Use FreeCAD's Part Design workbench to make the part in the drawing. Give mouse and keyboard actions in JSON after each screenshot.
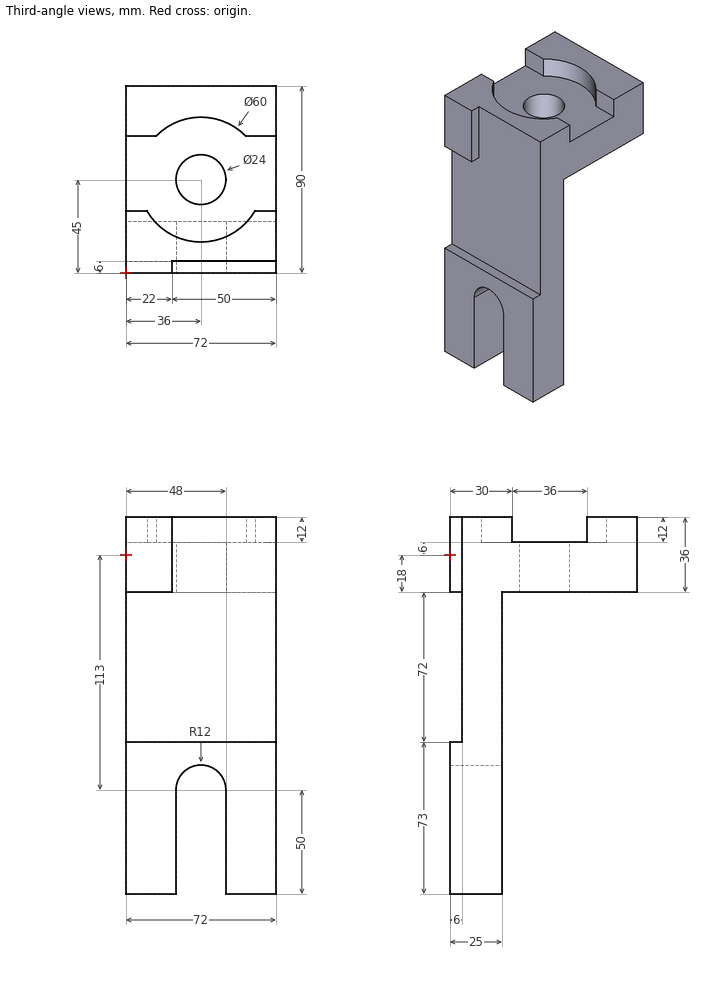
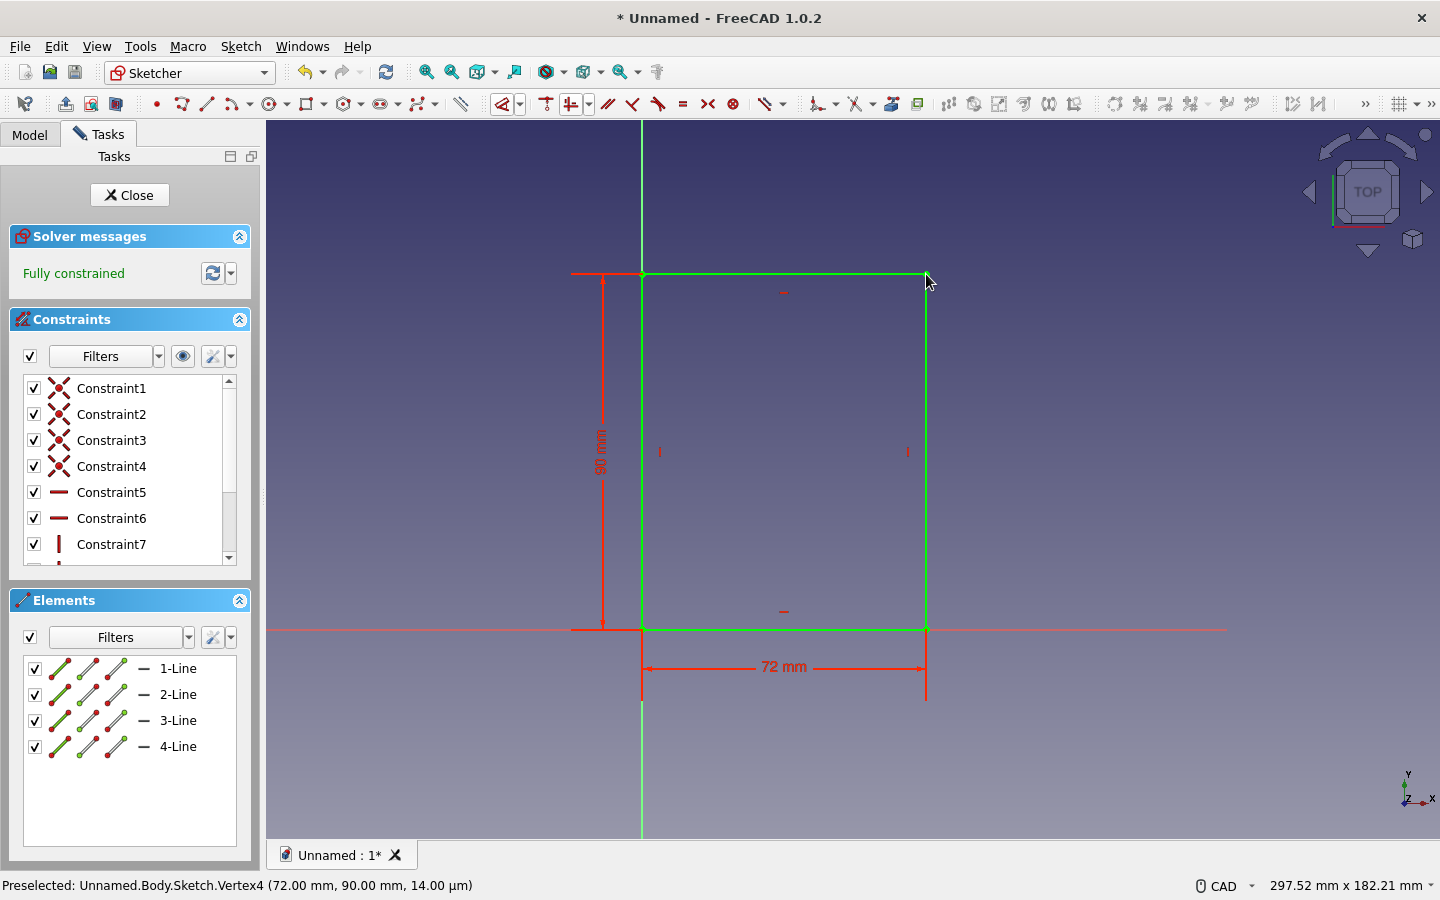
{"action": "left_click", "coordinate": [130, 195]}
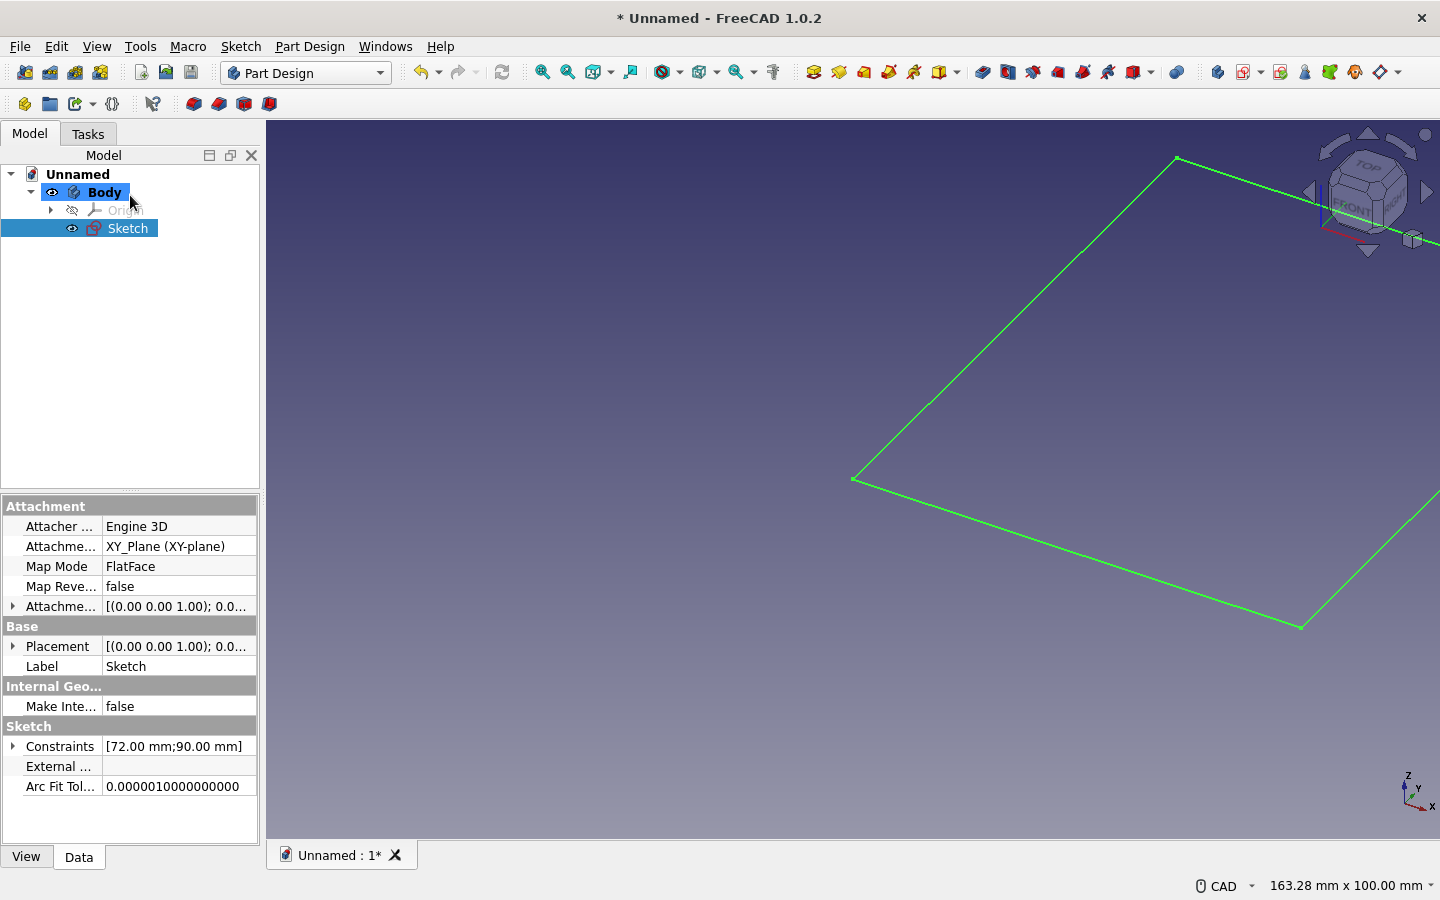
{"action": "left_click", "coordinate": [814, 72]}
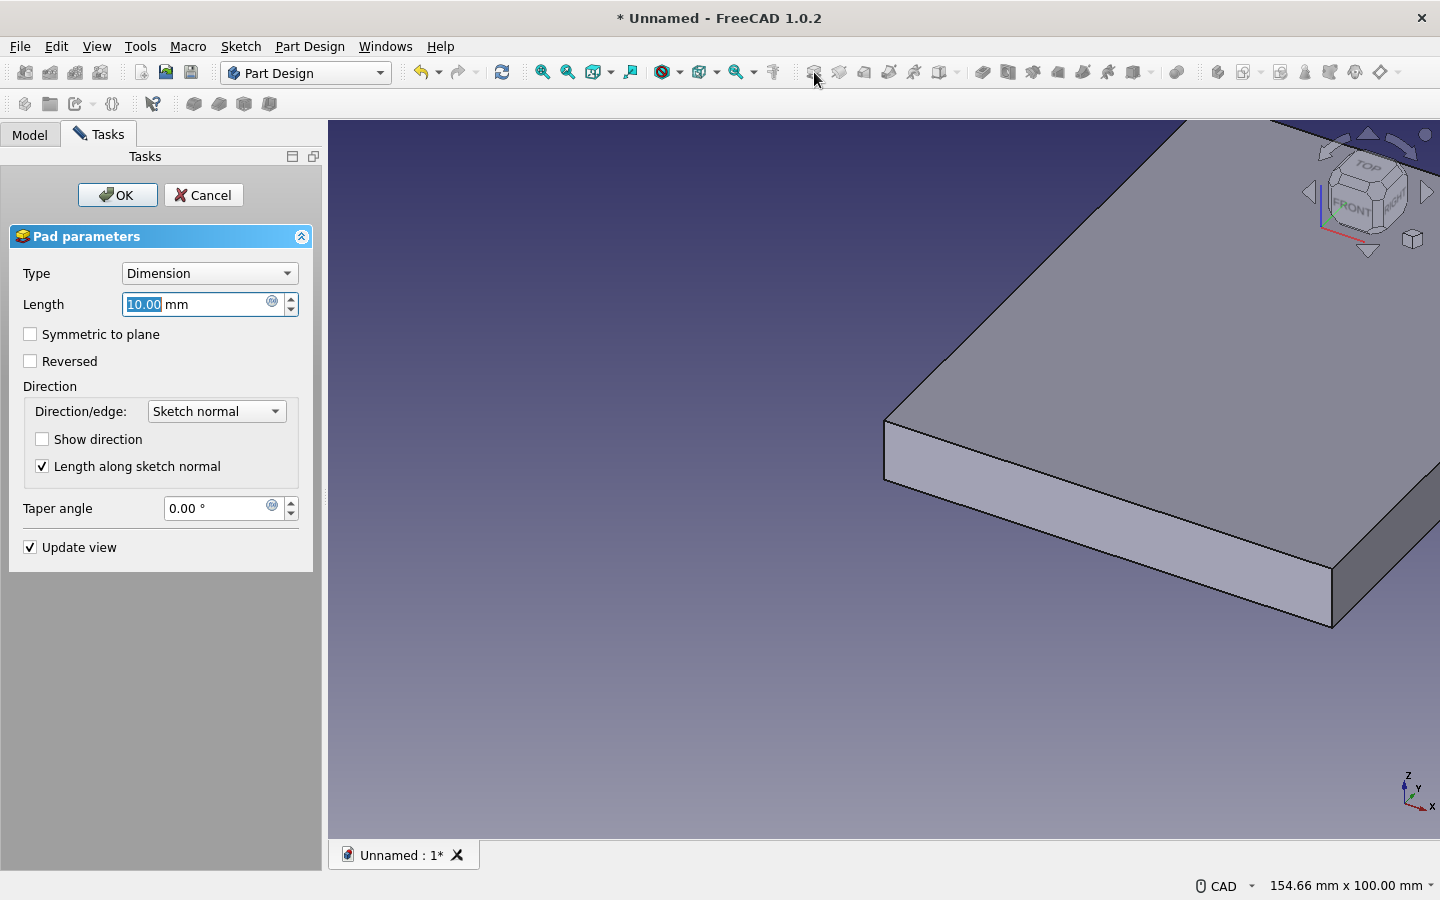
{"action": "type", "text": "36"}
{"action": "key", "text": "Tab"}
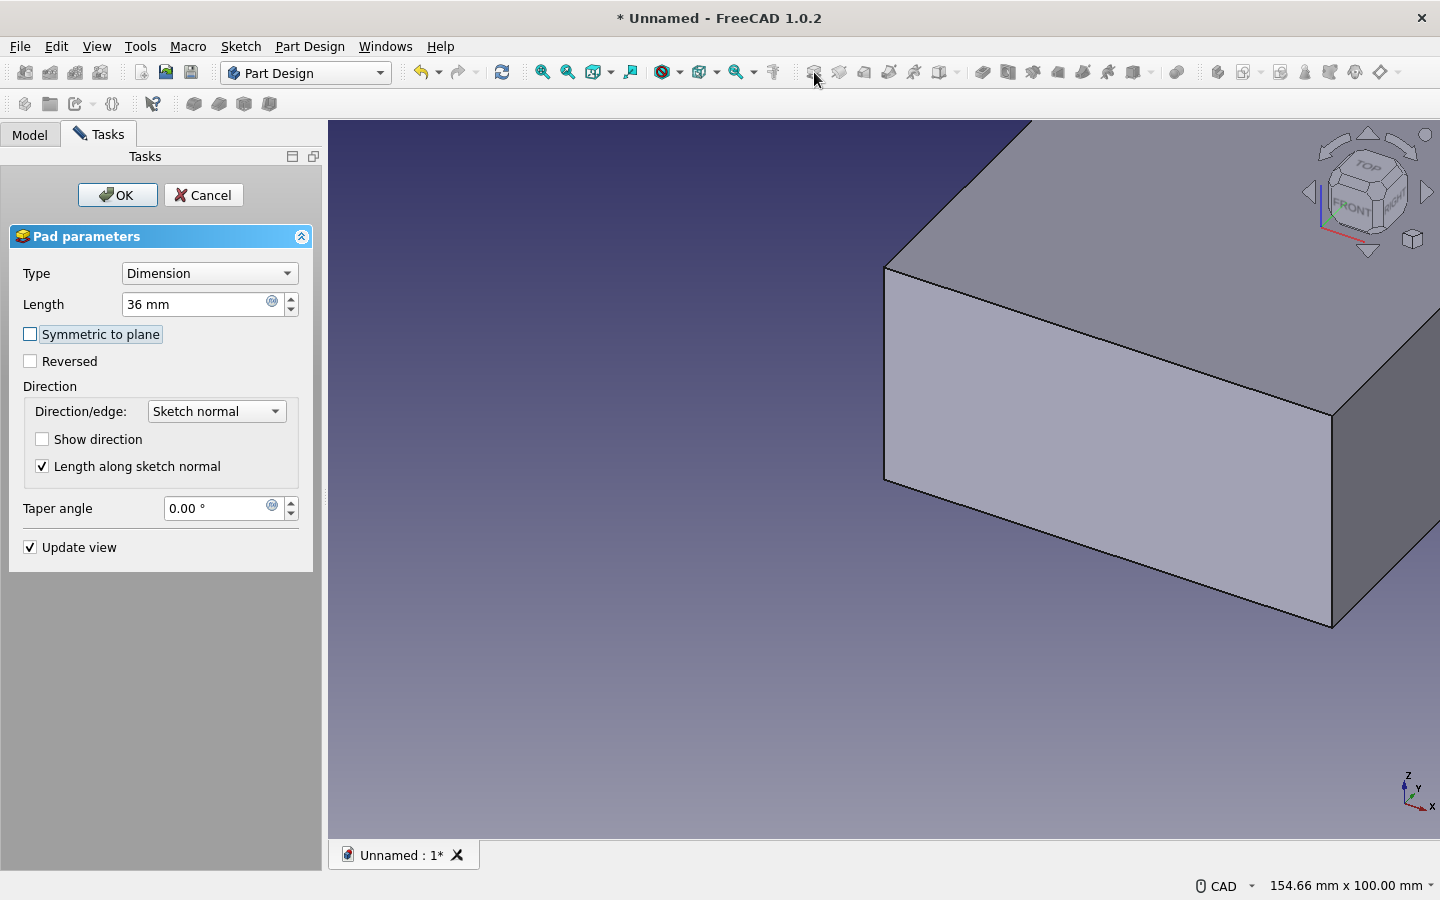
{"action": "left_click", "coordinate": [31, 334]}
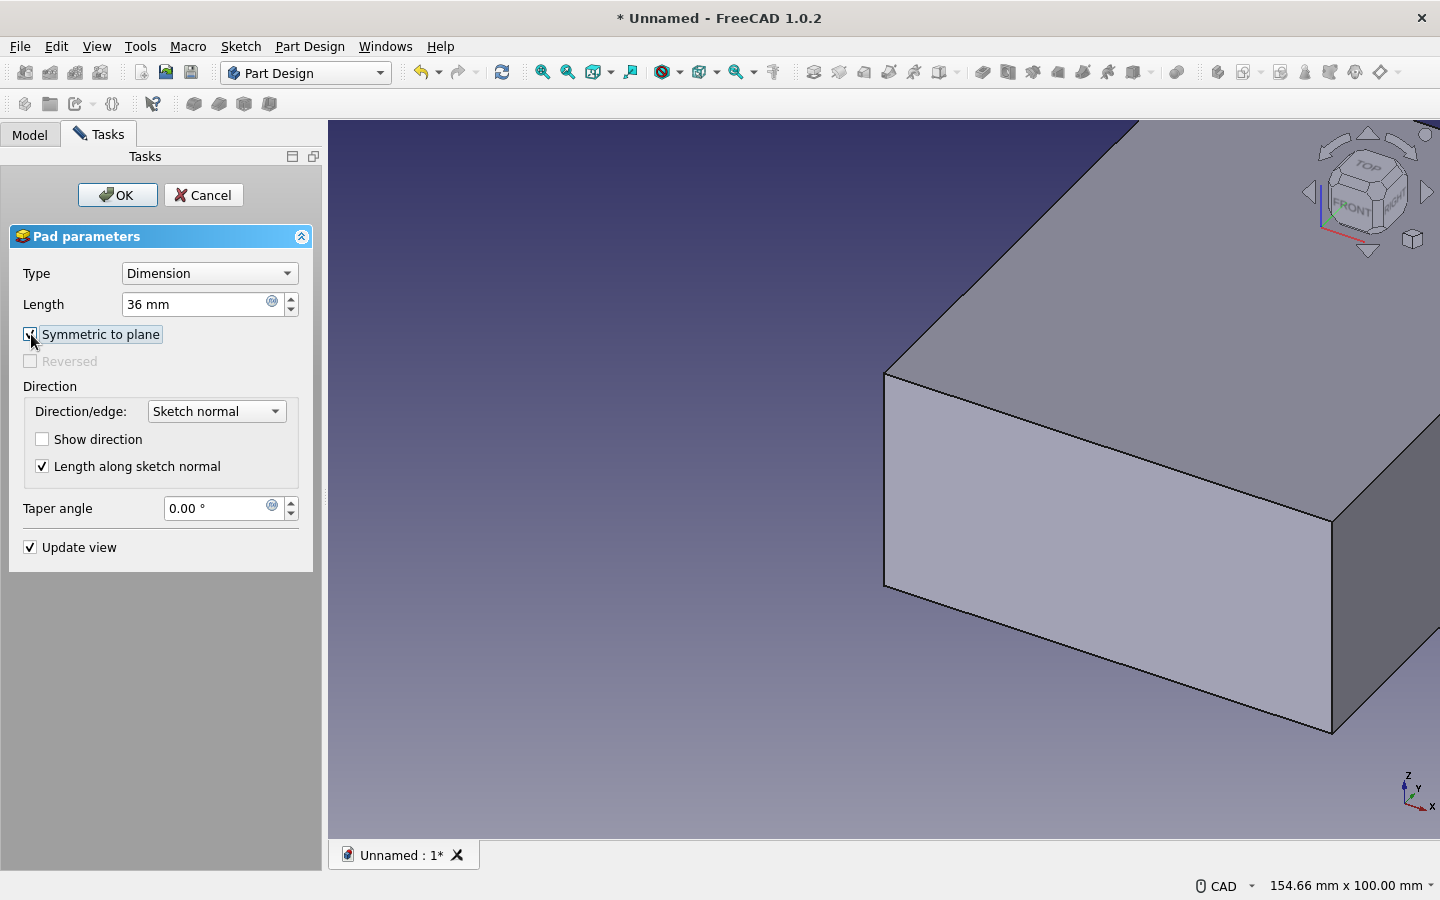
{"action": "left_click", "coordinate": [118, 195]}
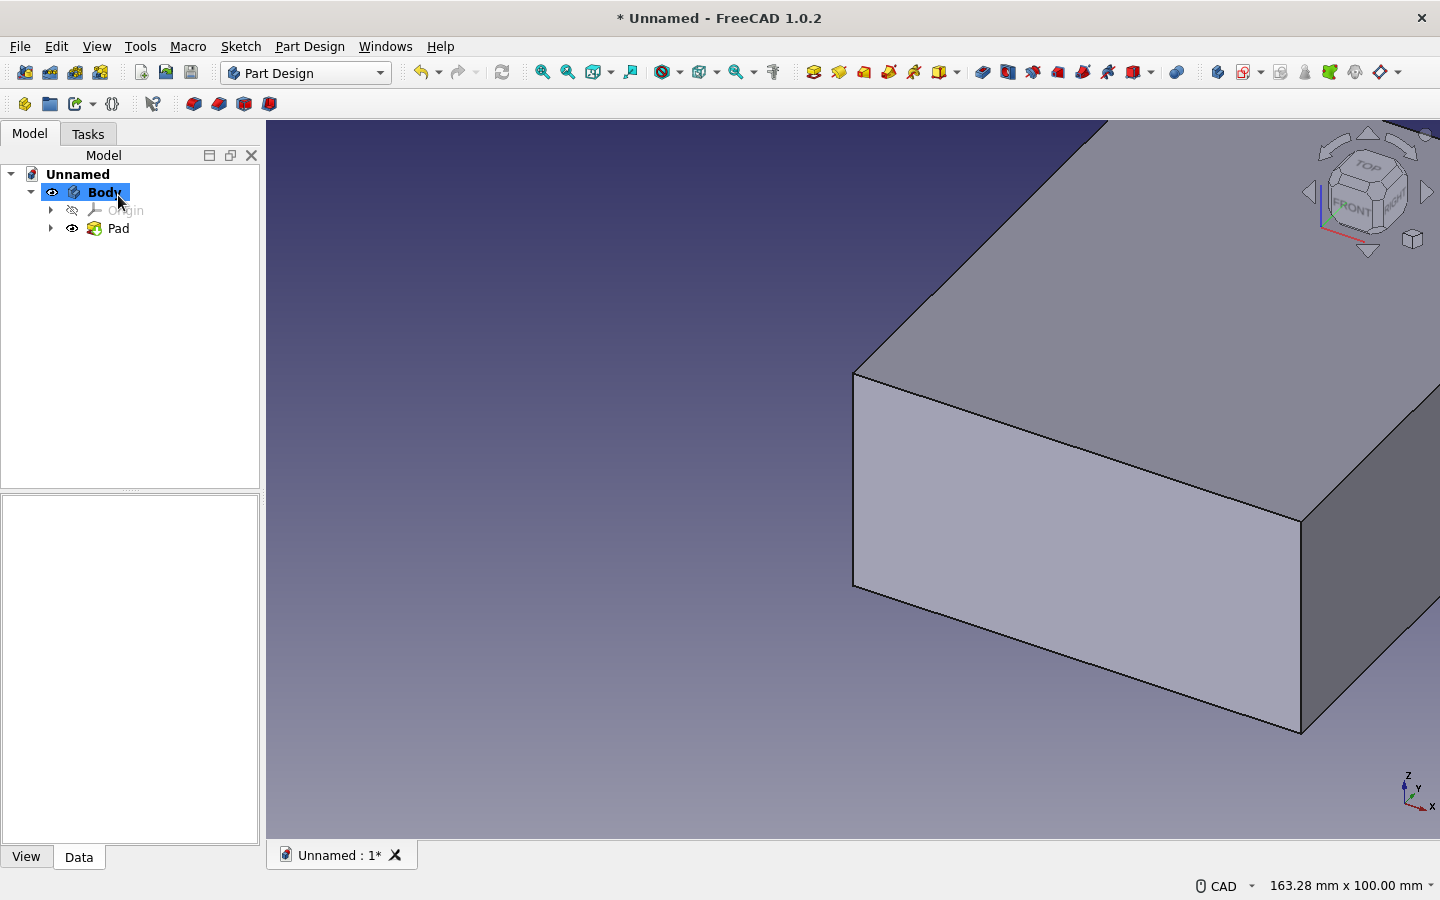
{"action": "key", "text": "v f"}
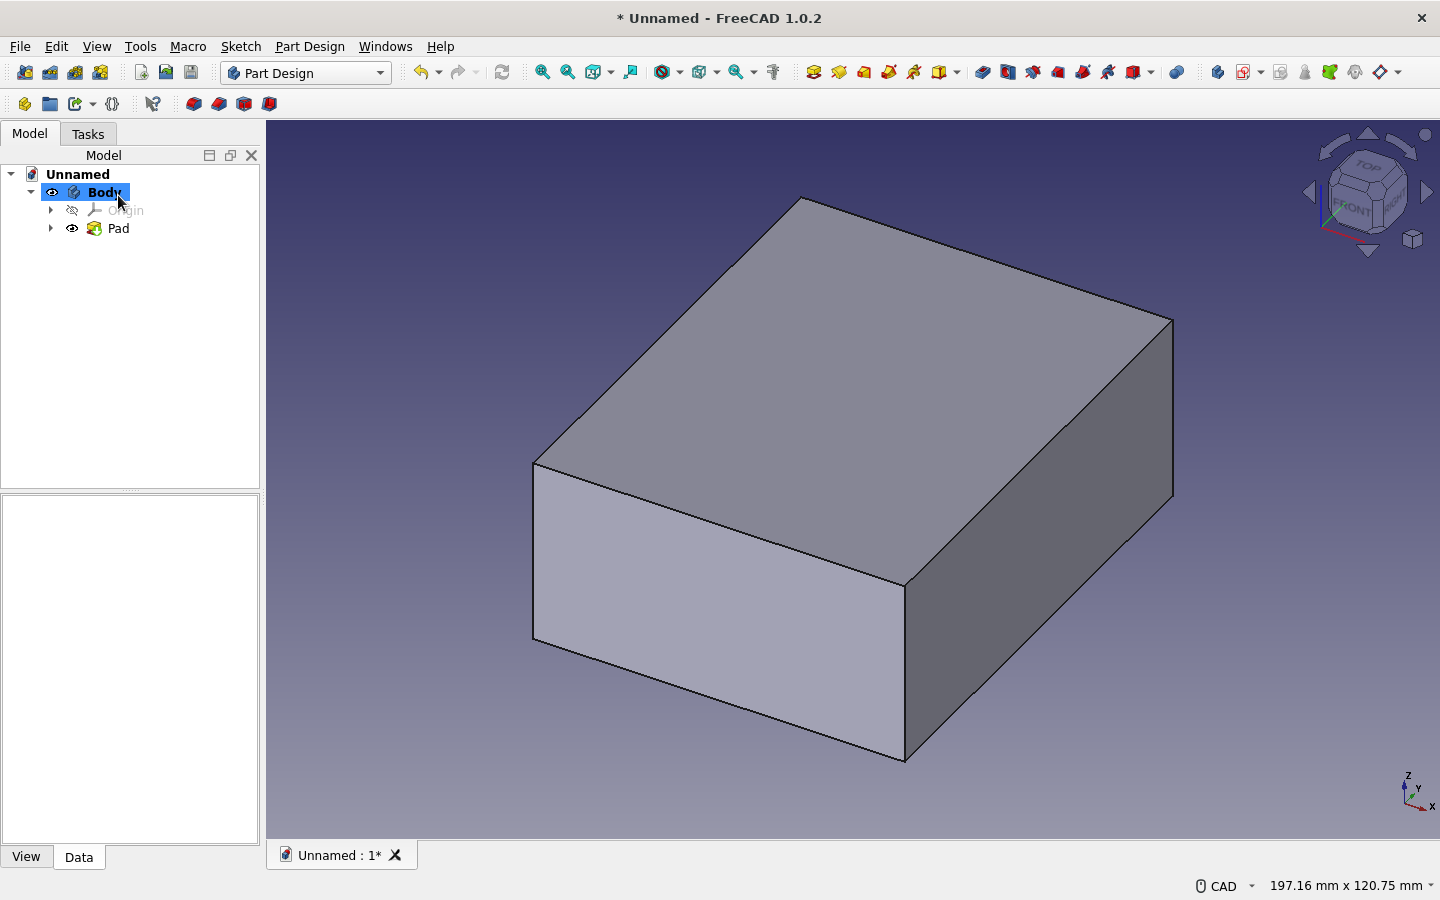
{"action": "left_click", "coordinate": [853, 391]}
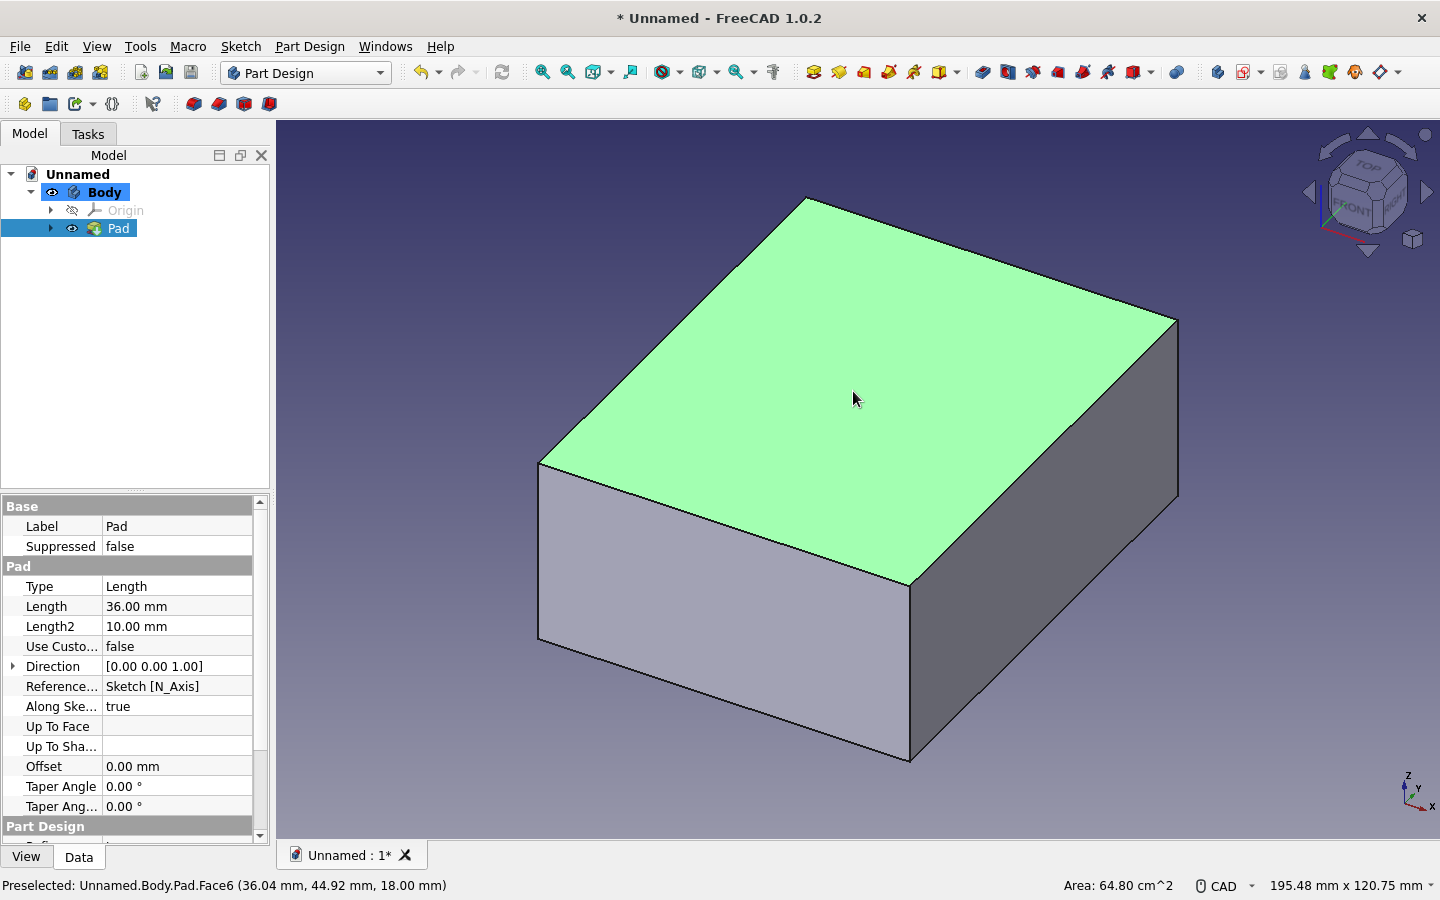
{"action": "left_click", "coordinate": [1242, 72]}